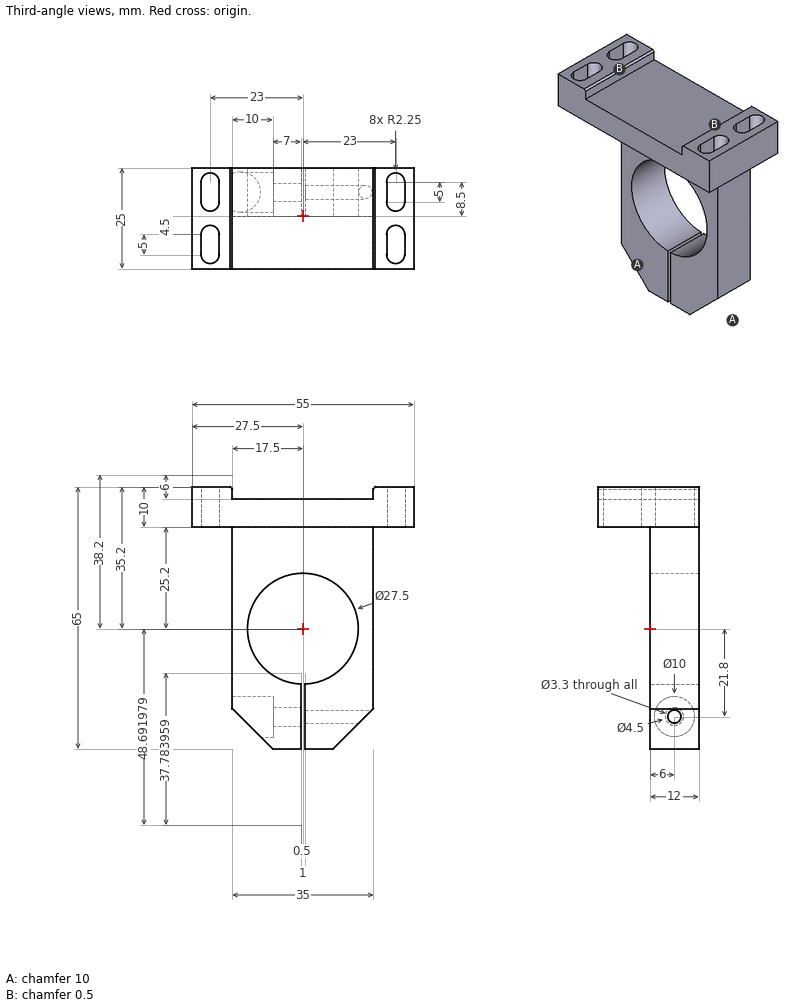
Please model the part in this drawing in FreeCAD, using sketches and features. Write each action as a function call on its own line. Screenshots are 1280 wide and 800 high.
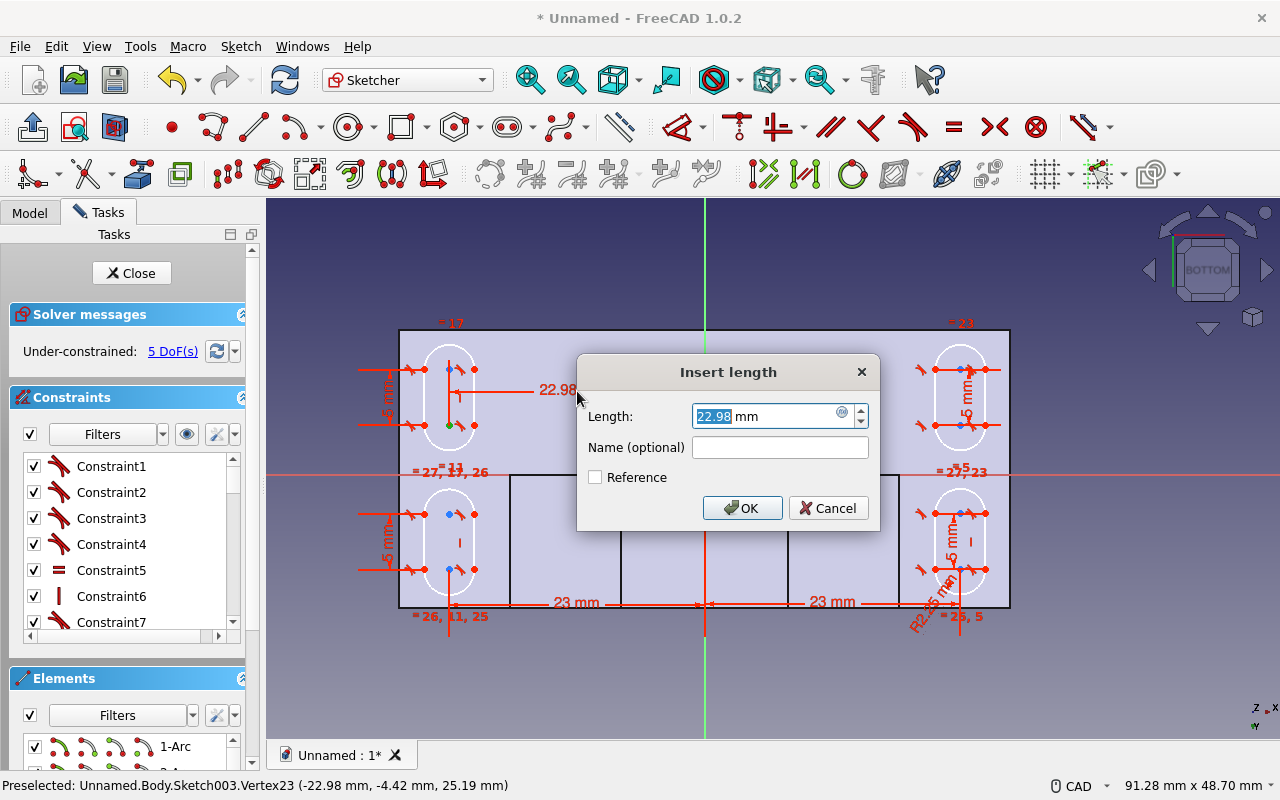
text(23)
key(Return)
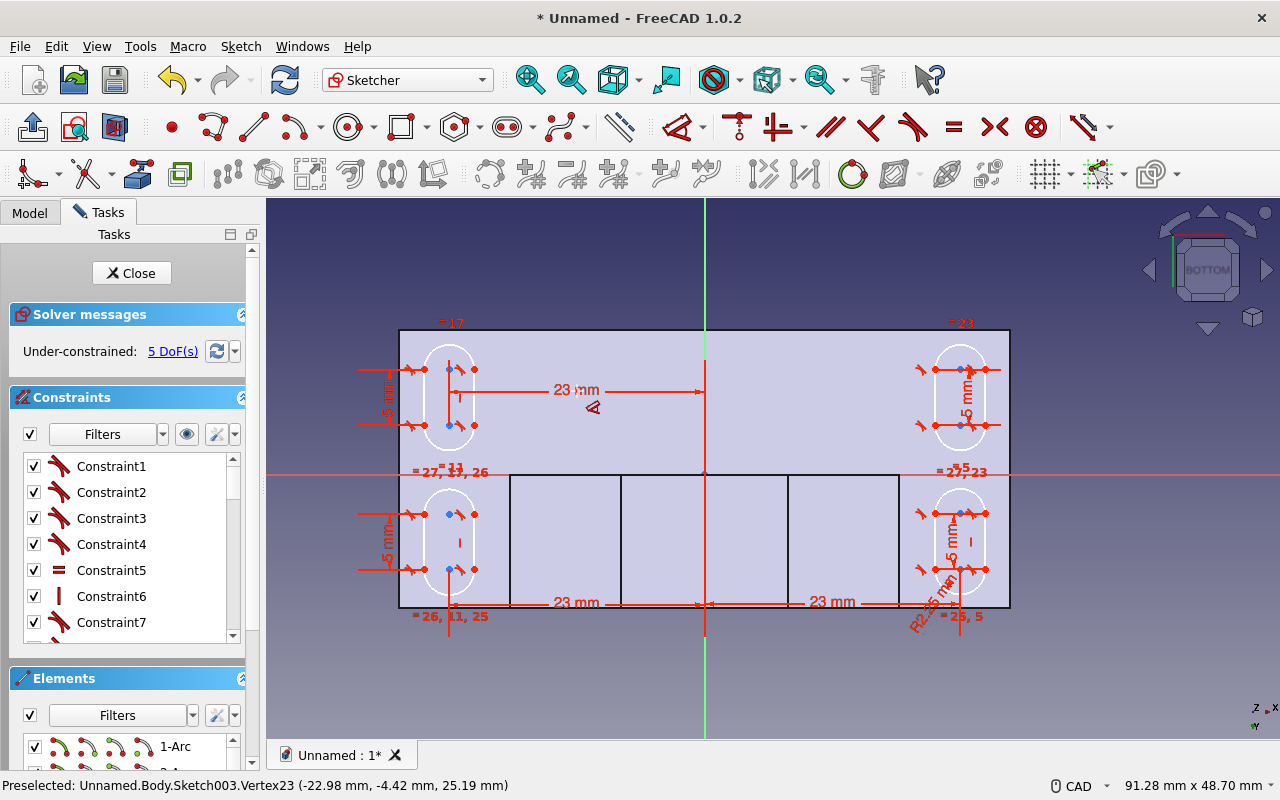
click(960, 425)
click(833, 391)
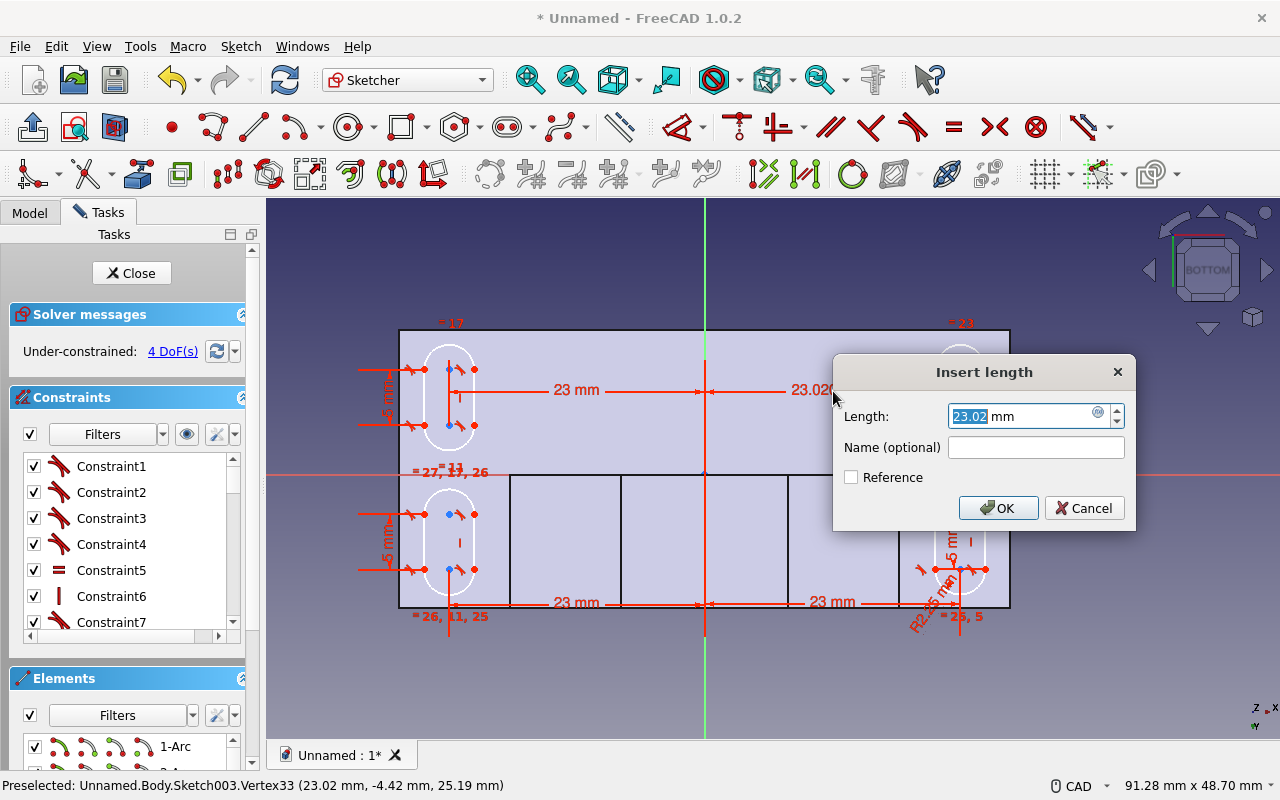
text(23)
key(Return)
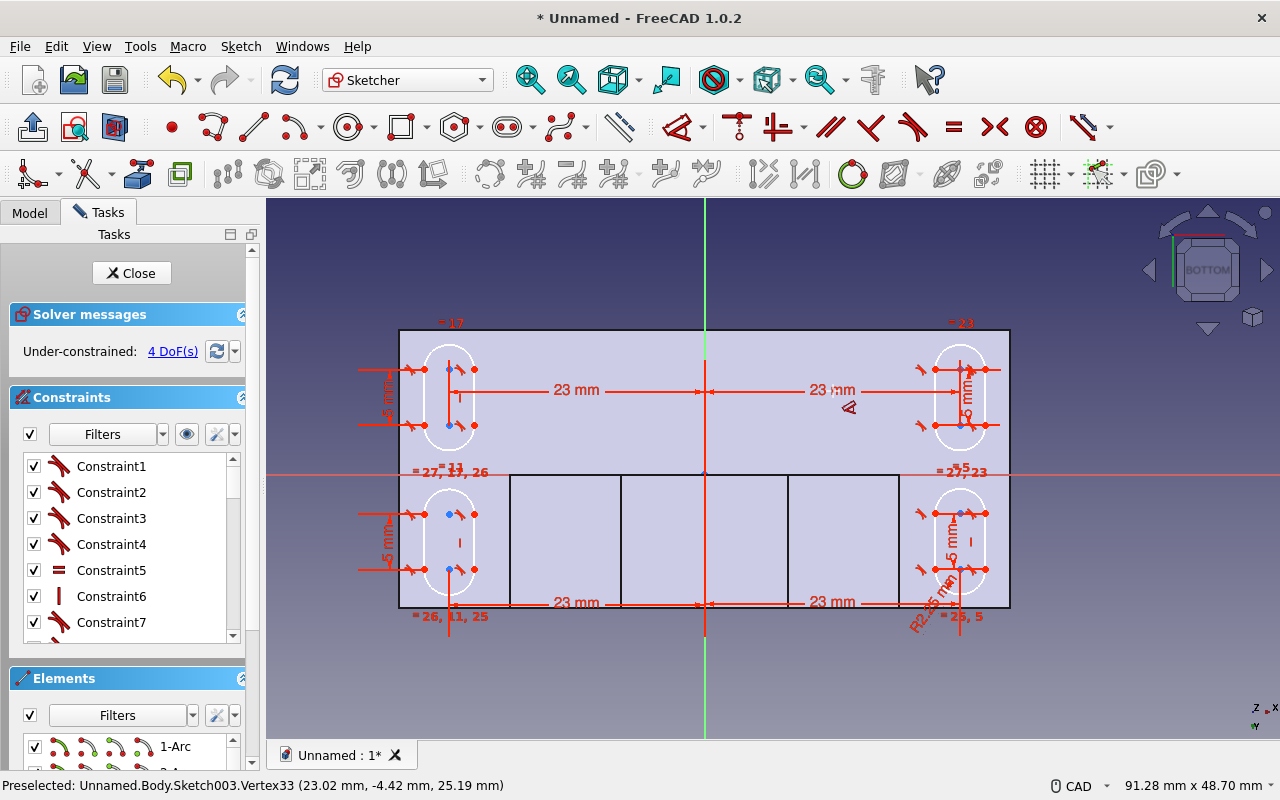
click(935, 569)
click(671, 522)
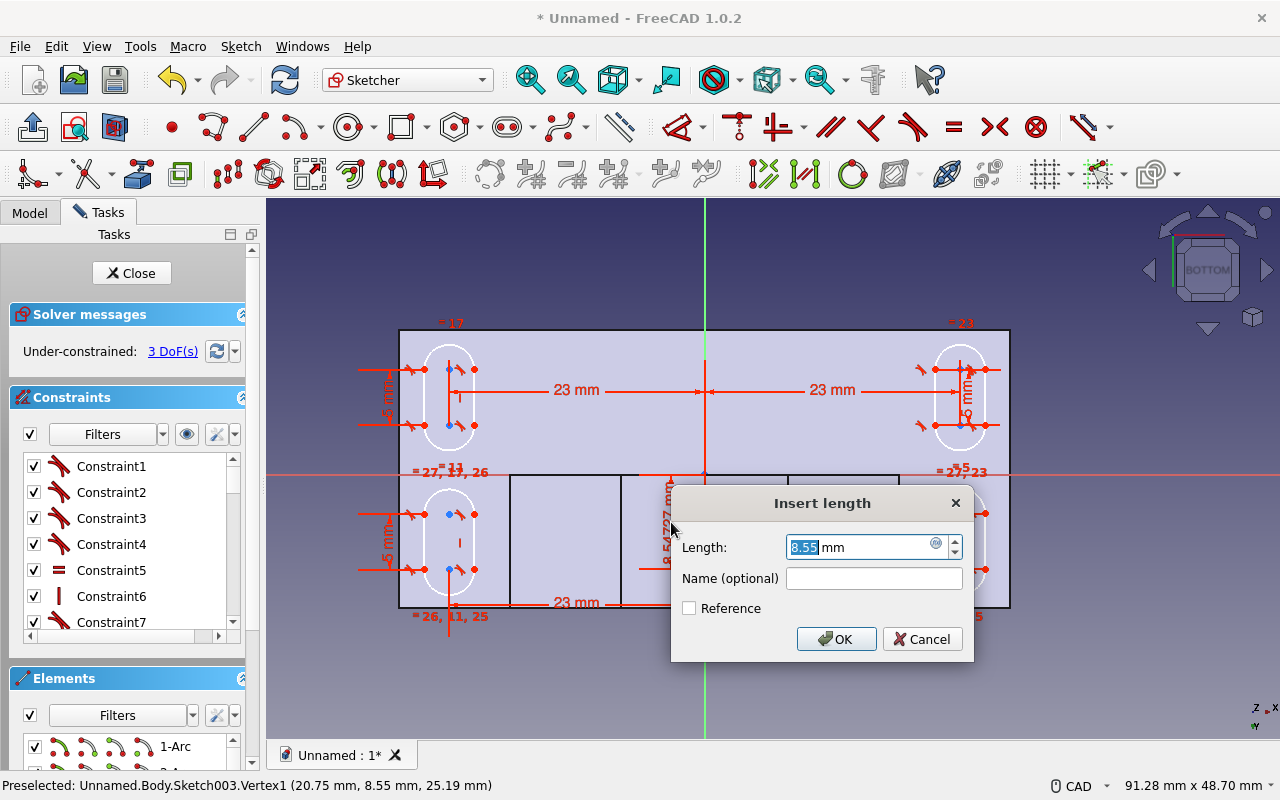
text(8.5)
key(Return)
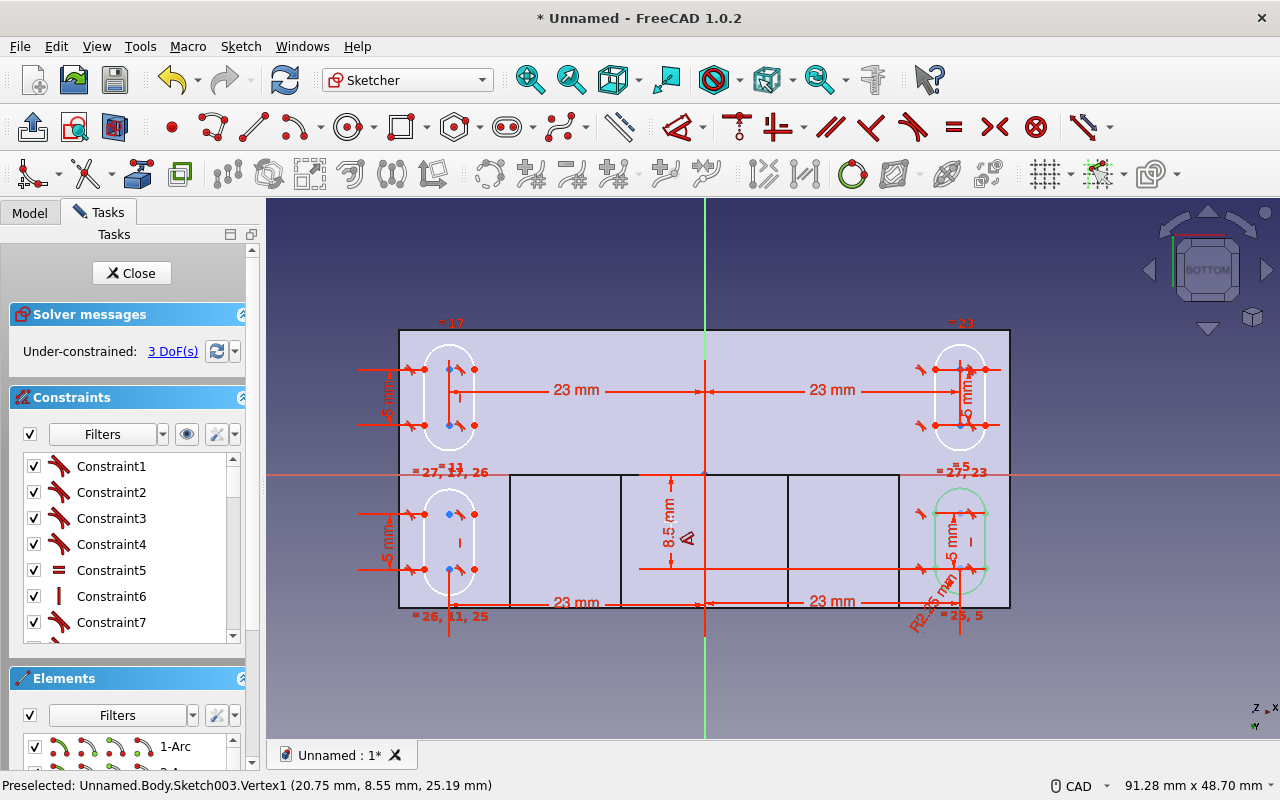
click(424, 570)
click(390, 500)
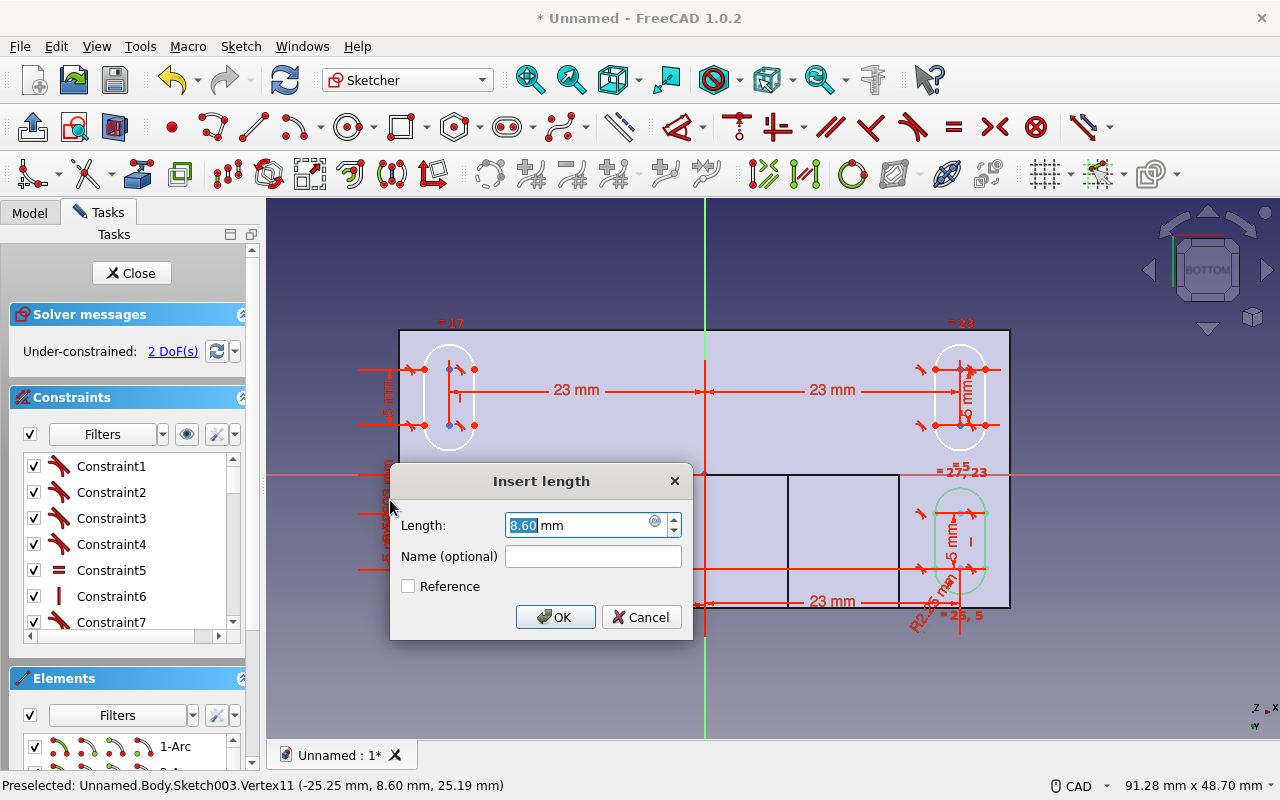
text(8.5)
key(Return)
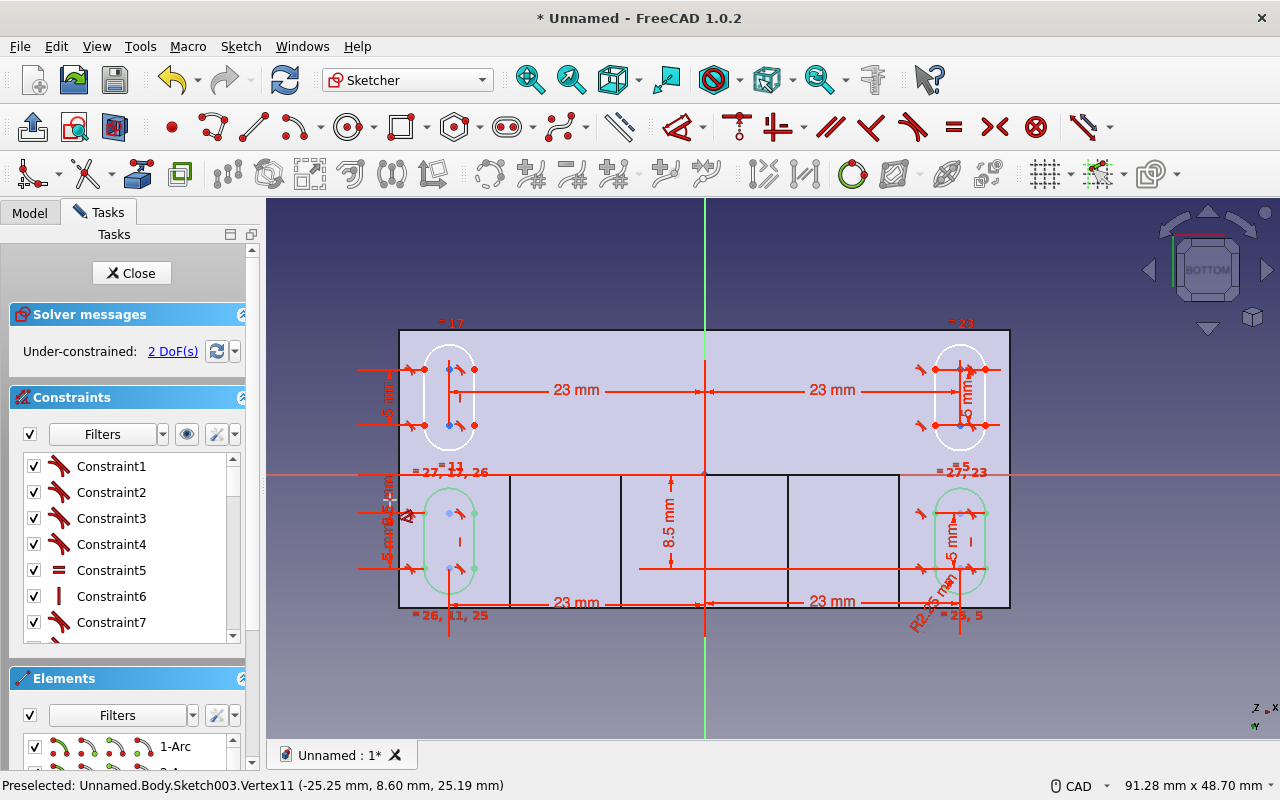
click(424, 425)
click(390, 450)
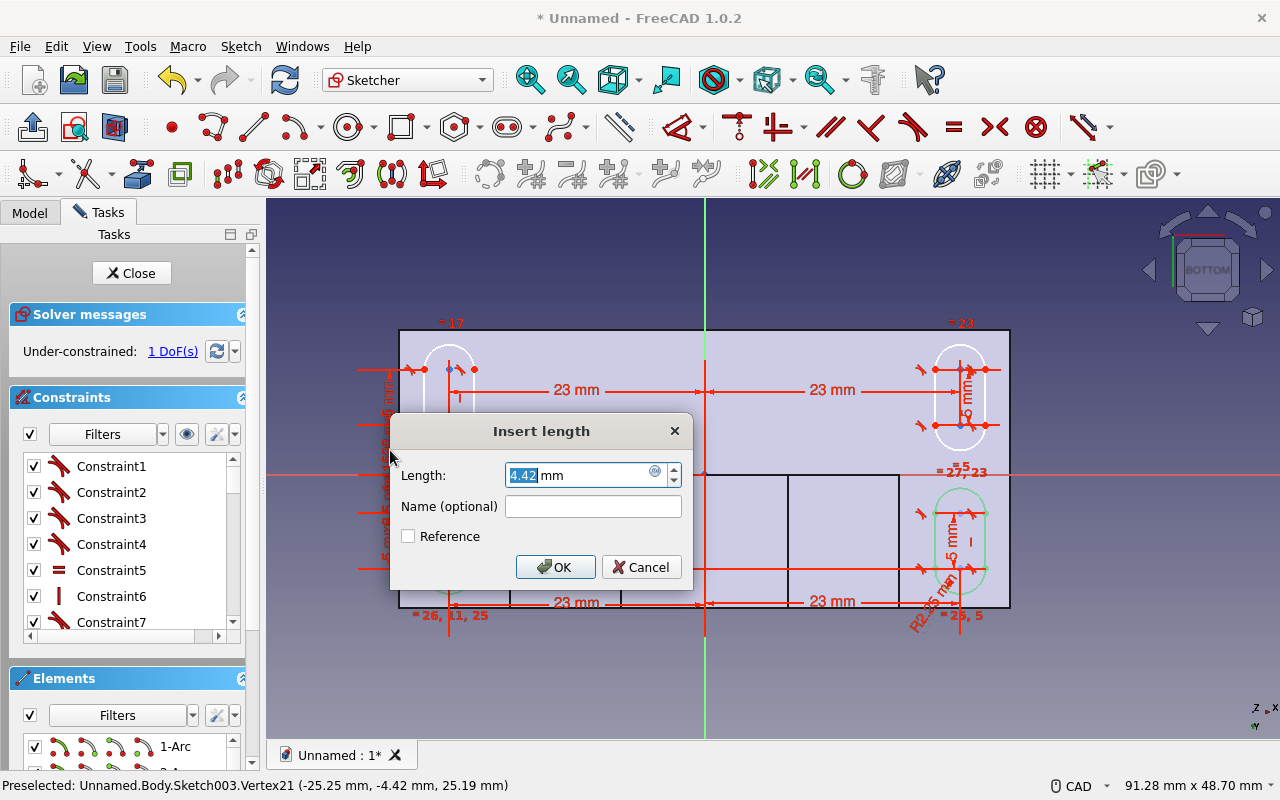
text(4.5)
key(Return)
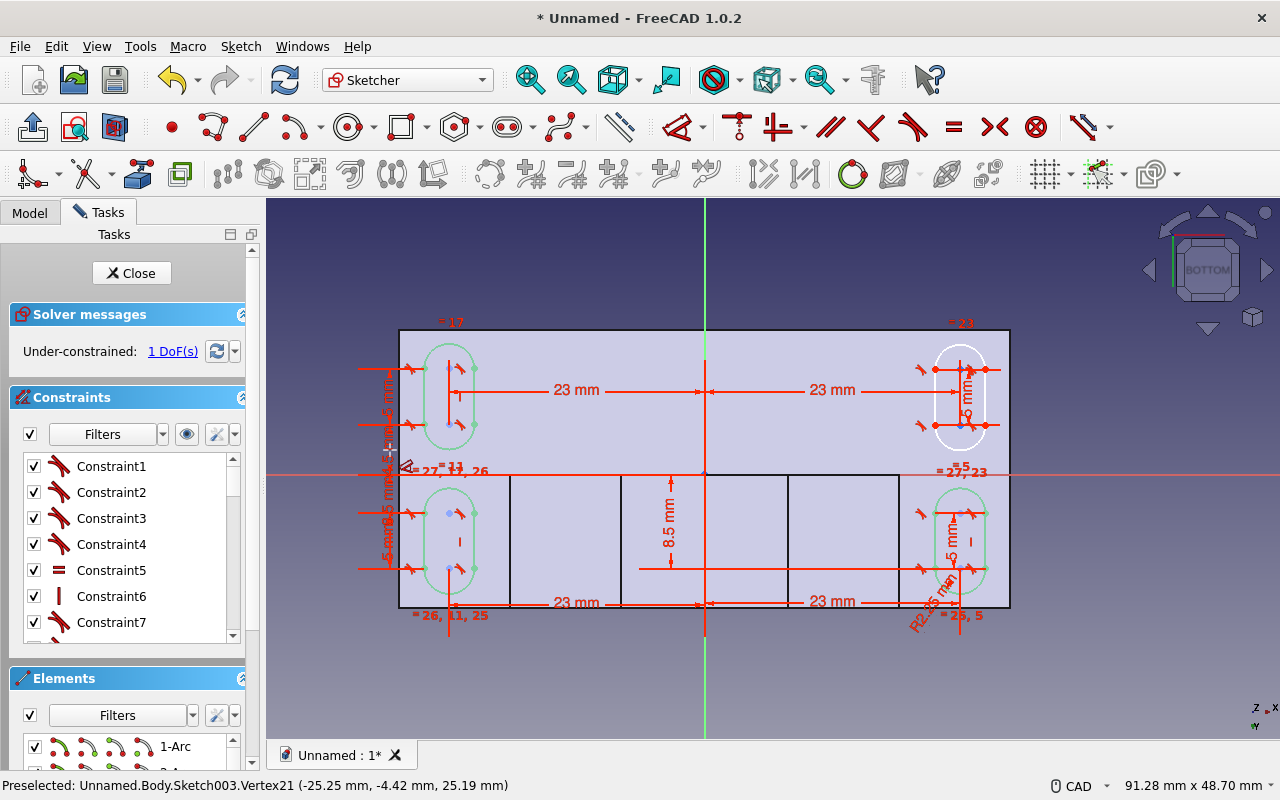
click(935, 425)
click(969, 433)